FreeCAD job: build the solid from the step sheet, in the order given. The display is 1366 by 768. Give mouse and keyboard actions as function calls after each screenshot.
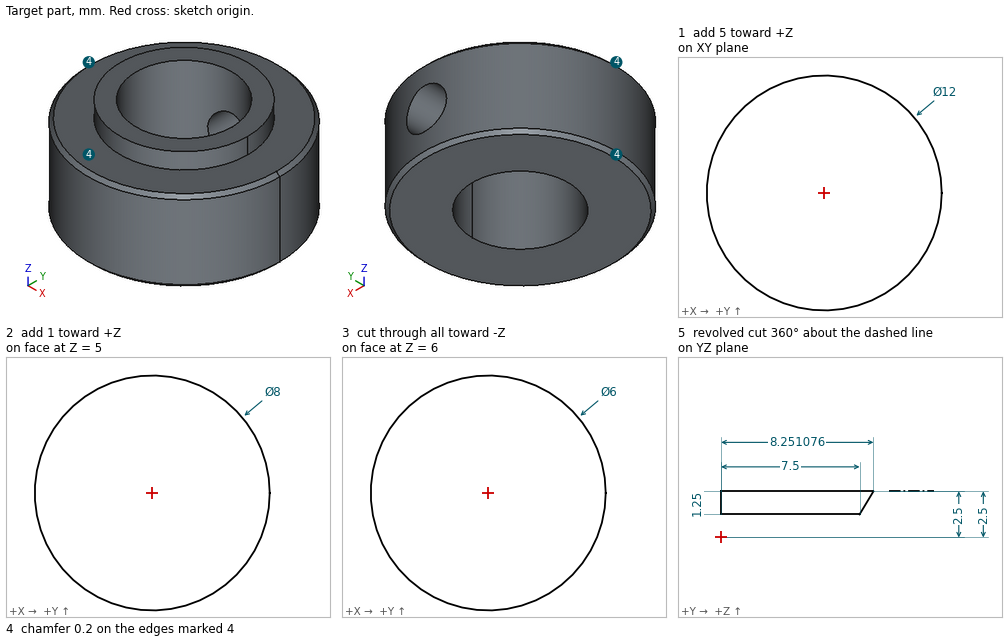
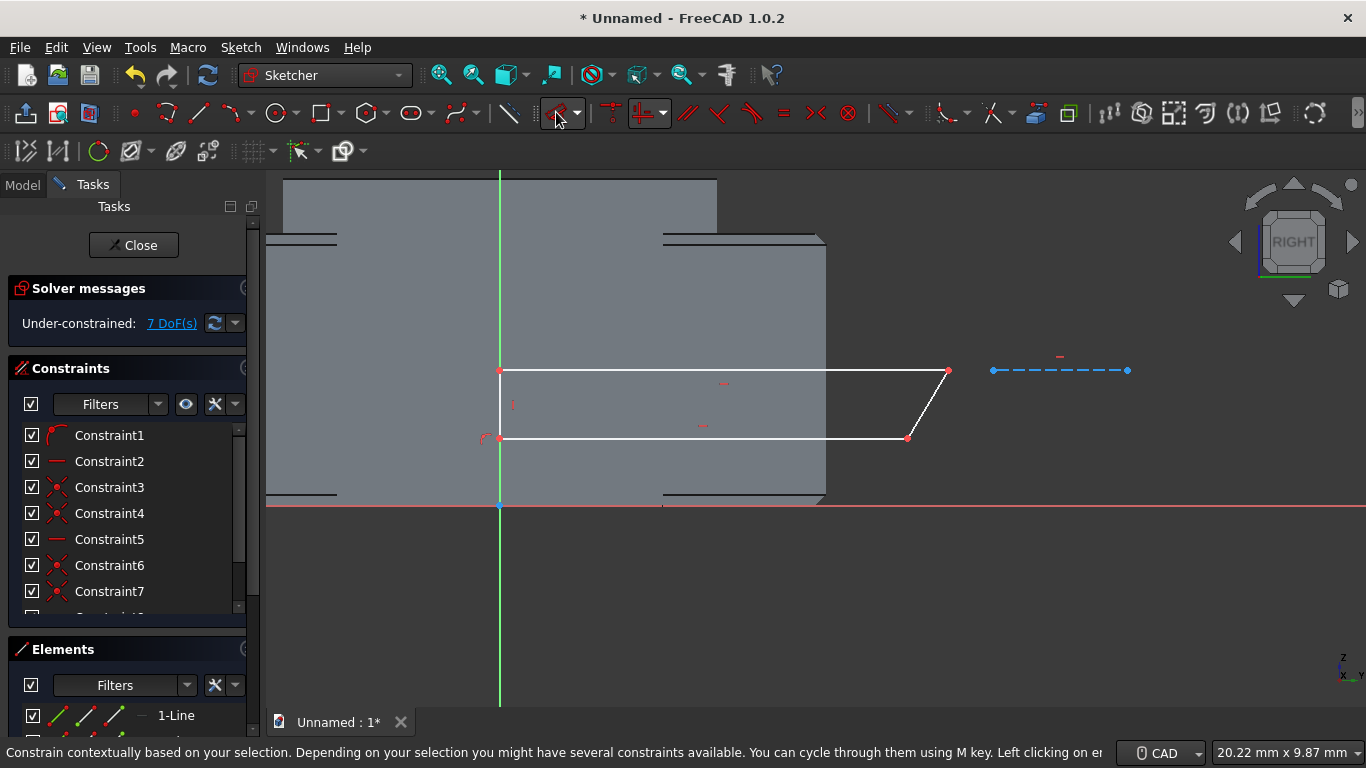
click(622, 439)
click(704, 473)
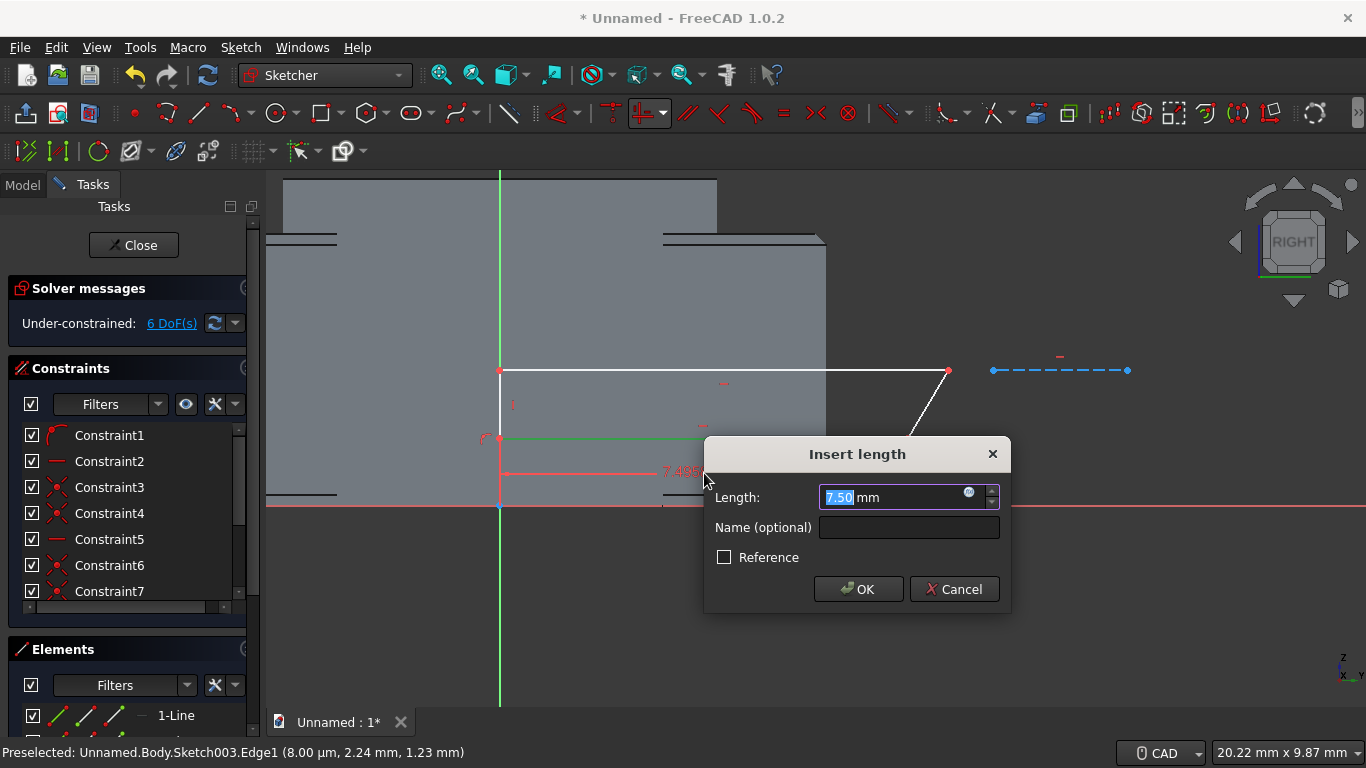
text(7.5)
key(Return)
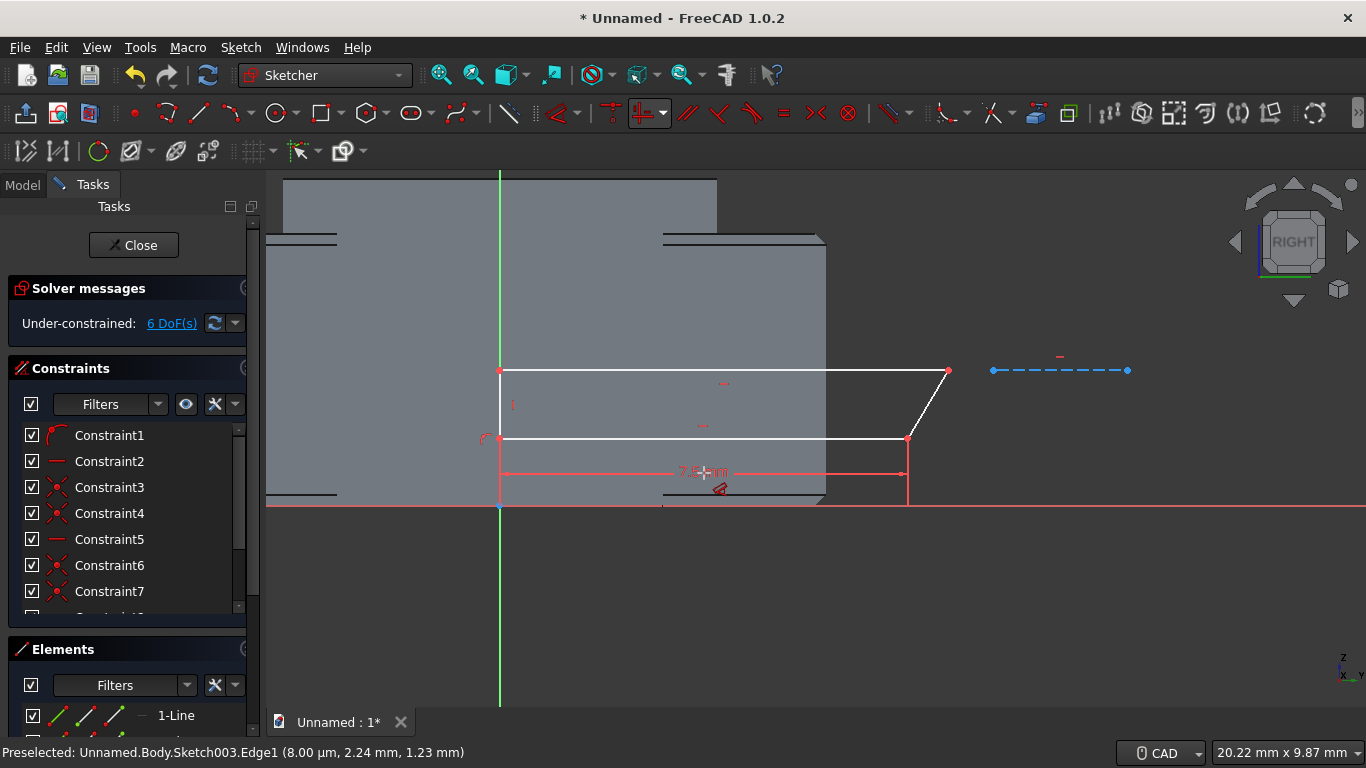
click(500, 391)
click(466, 405)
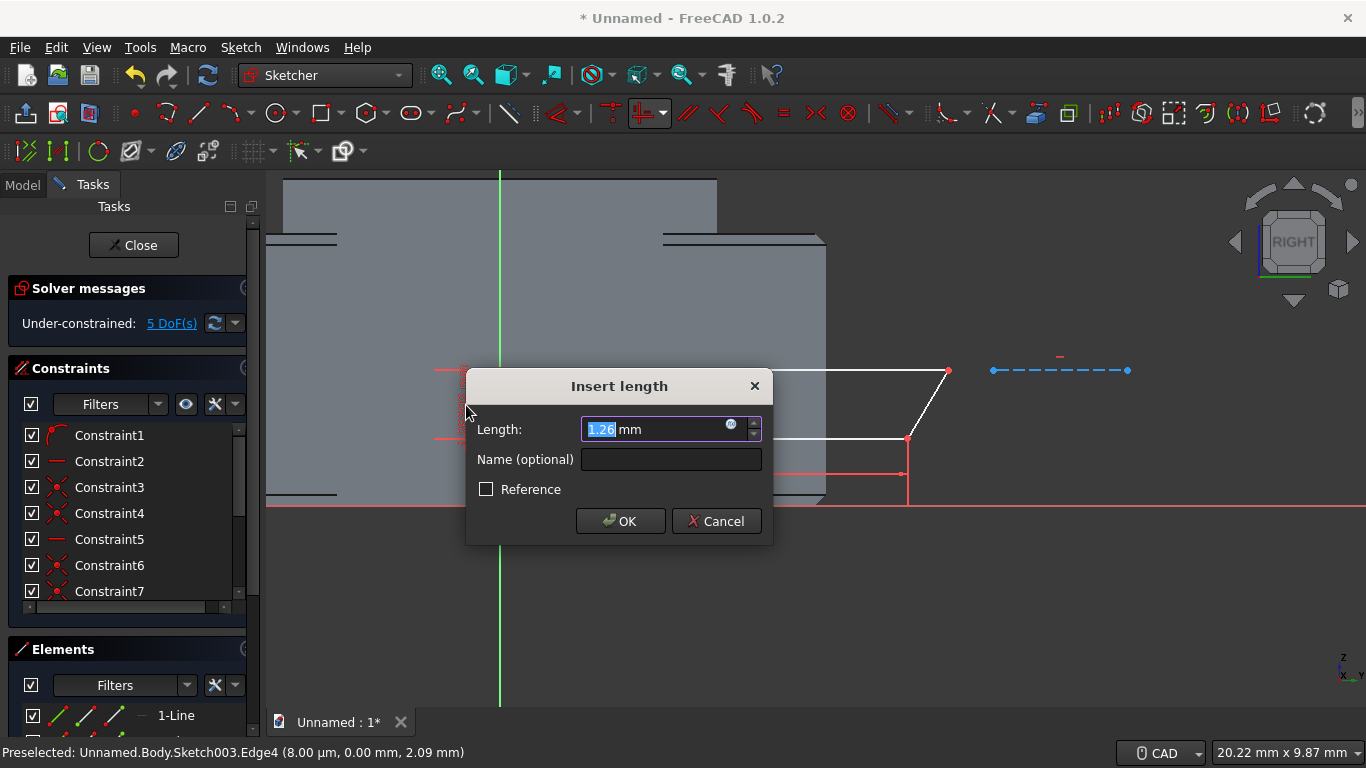
text(1.25)
key(Return)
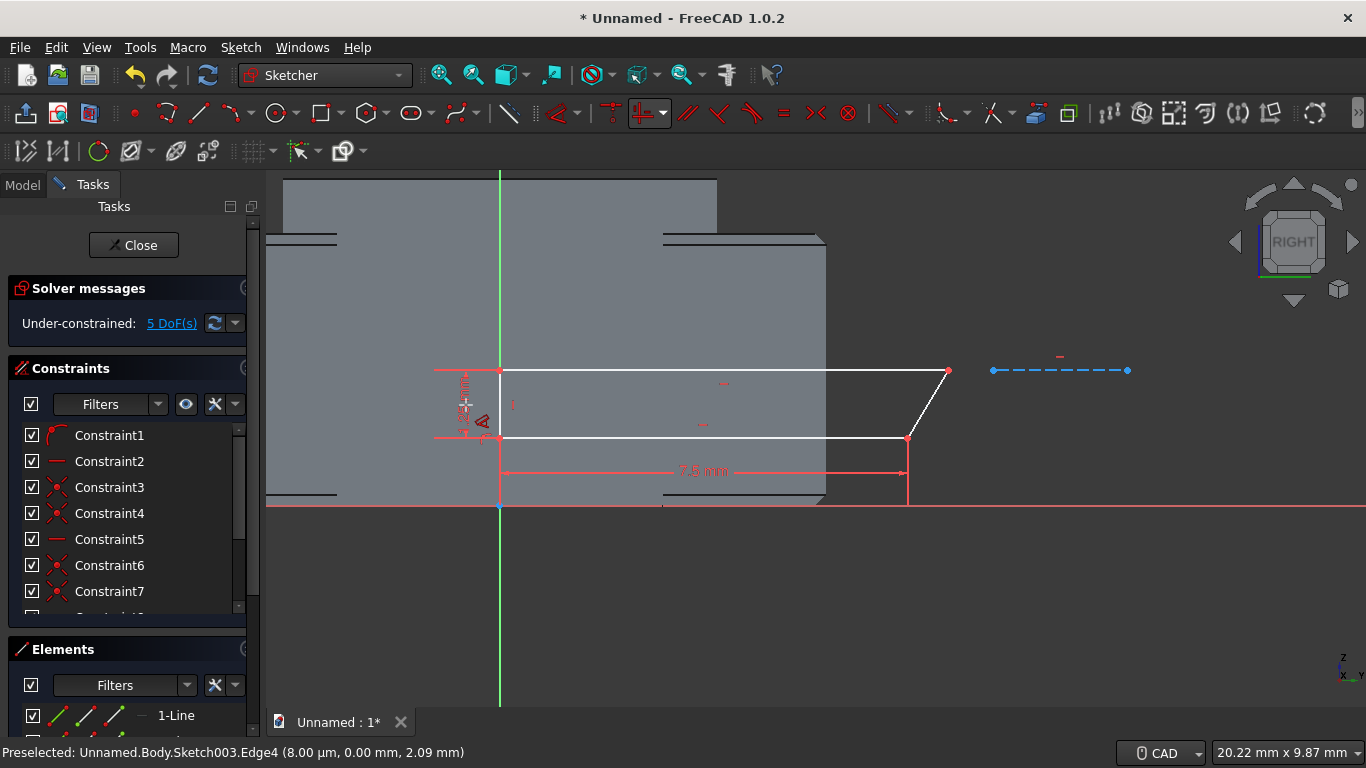
click(949, 370)
click(466, 438)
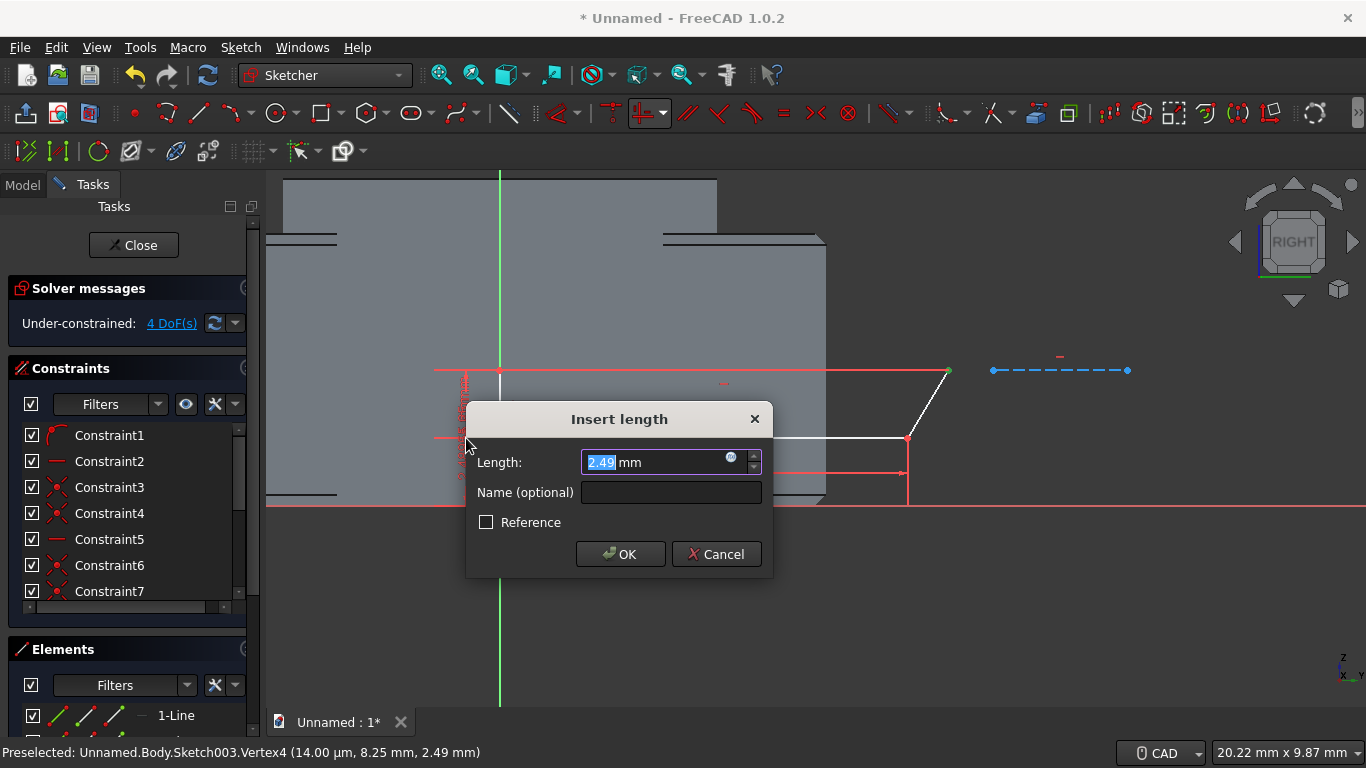
text(2.5)
key(Return)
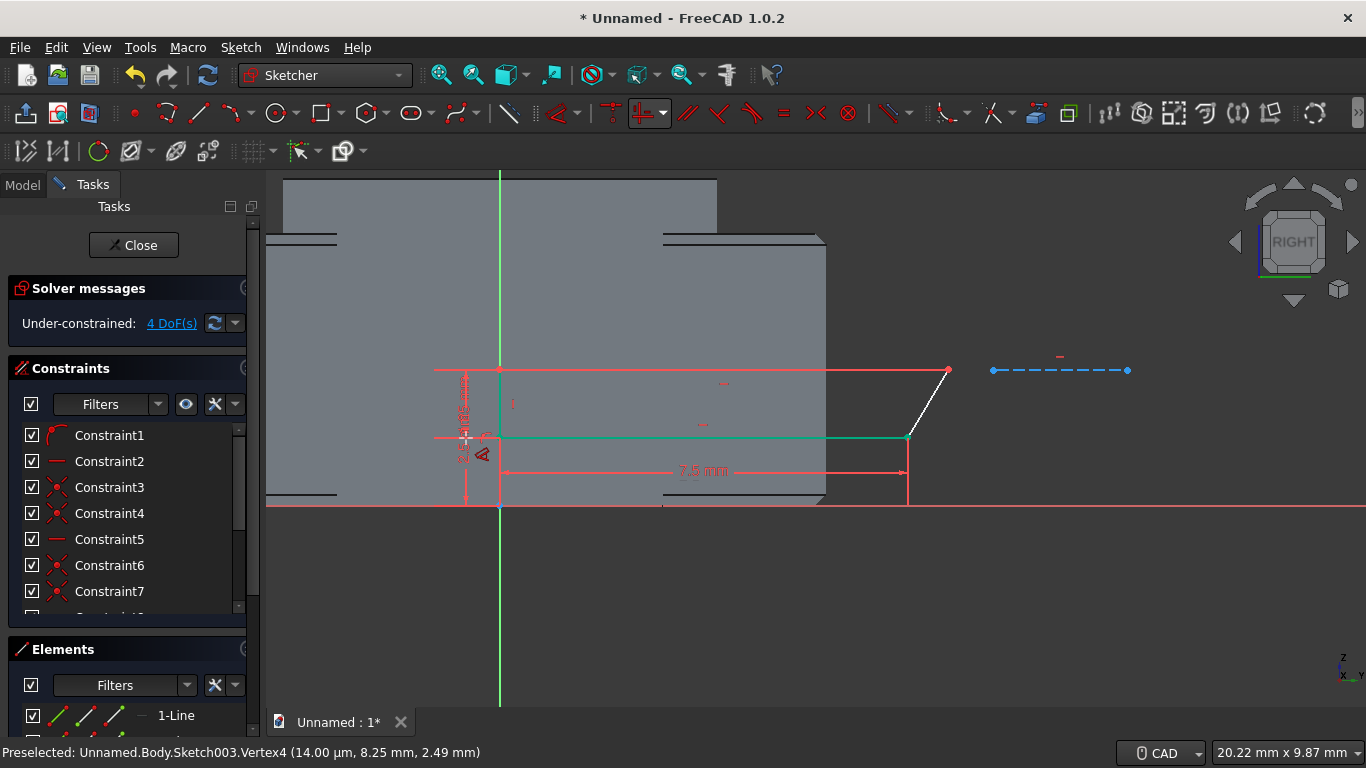
click(993, 370)
click(466, 469)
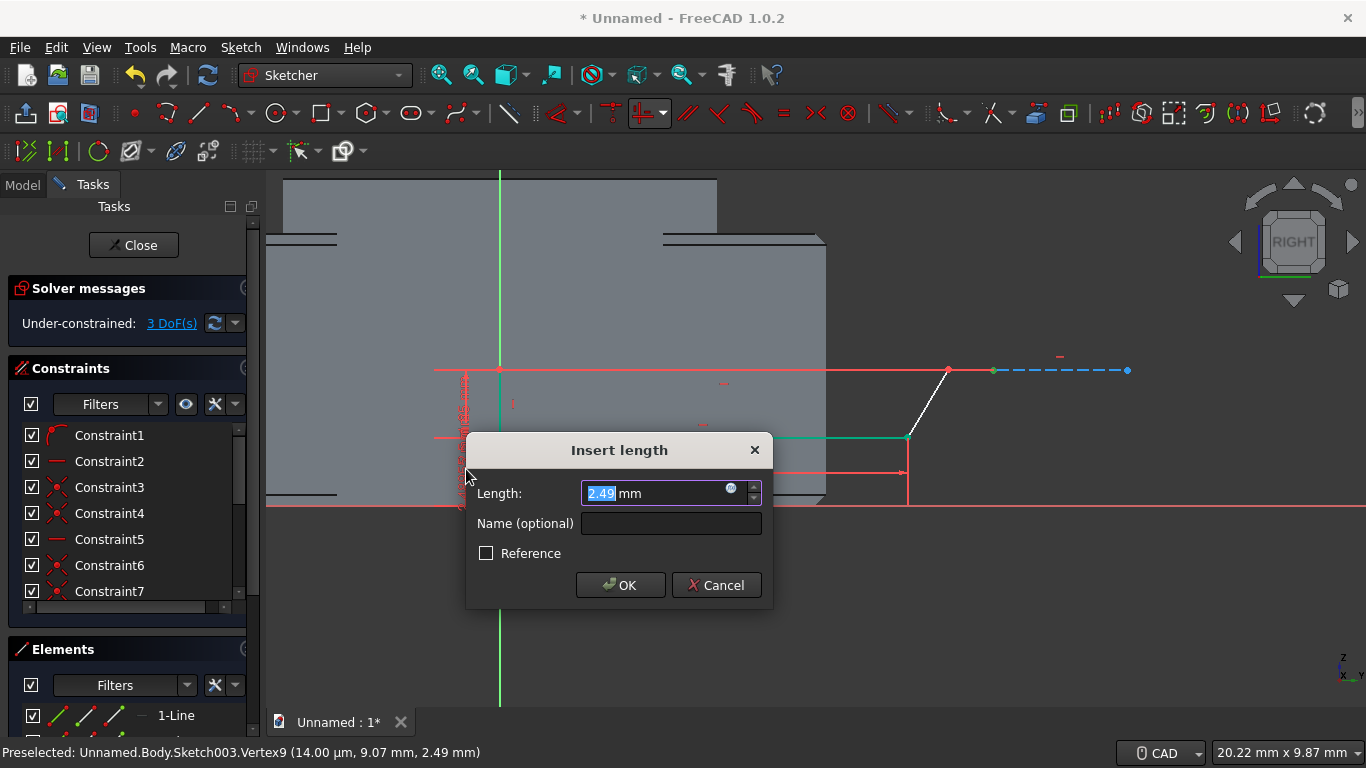
text(2.5)
key(Return)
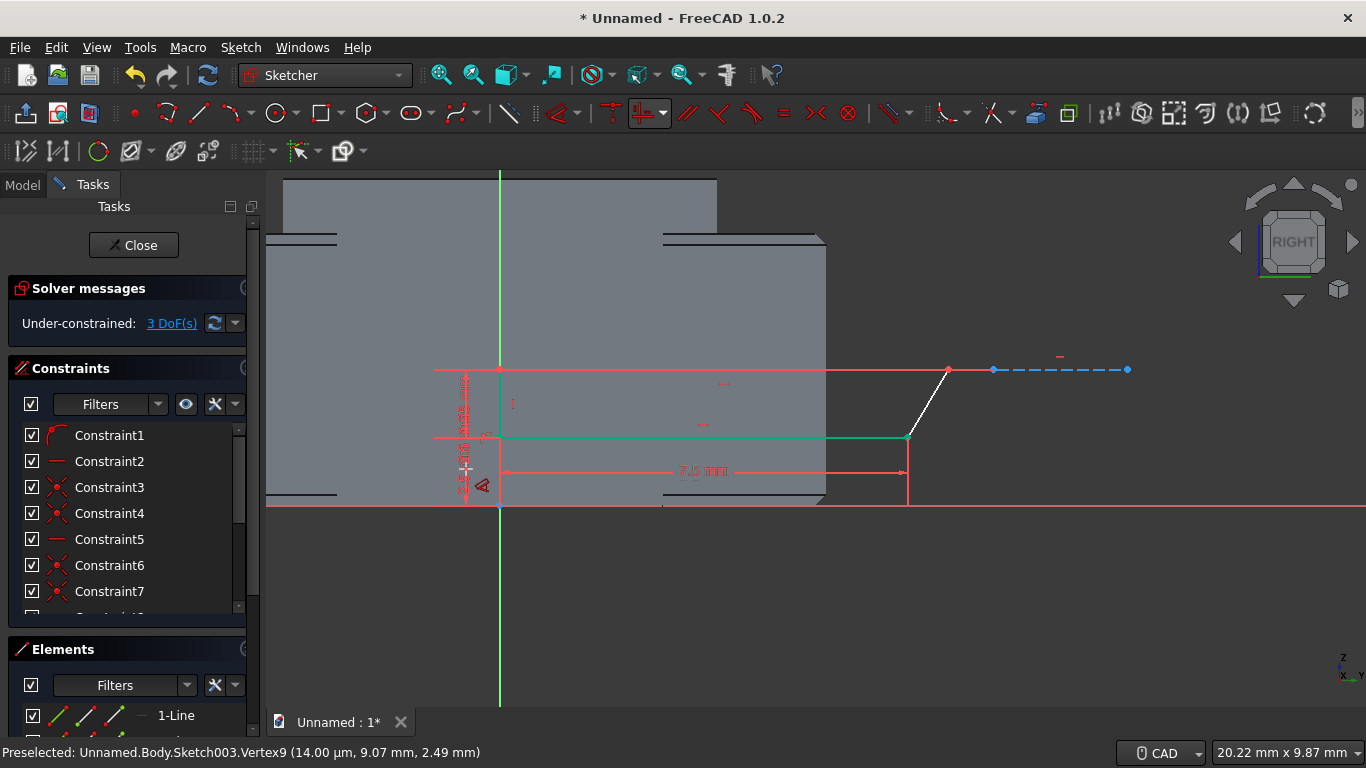
click(814, 370)
click(724, 336)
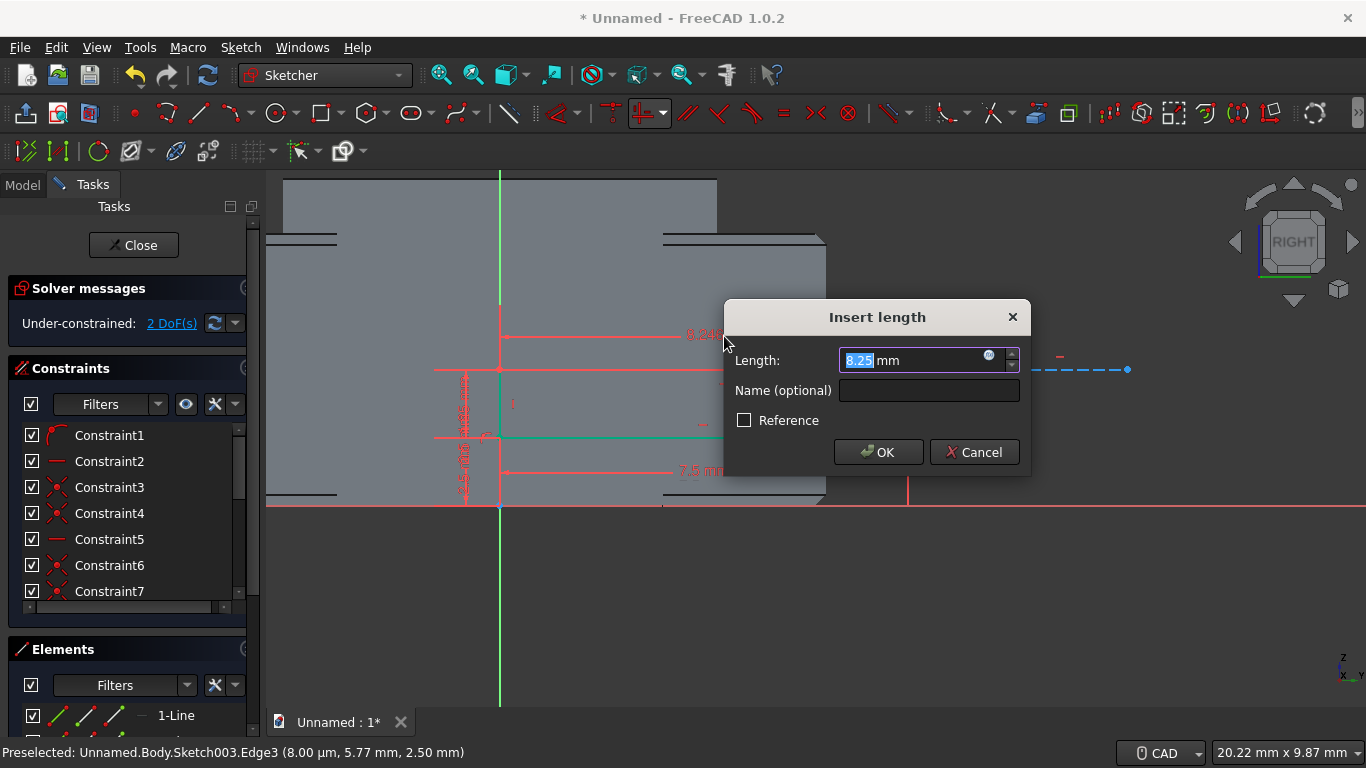
text(8.251076)
key(Return)
key(Escape)